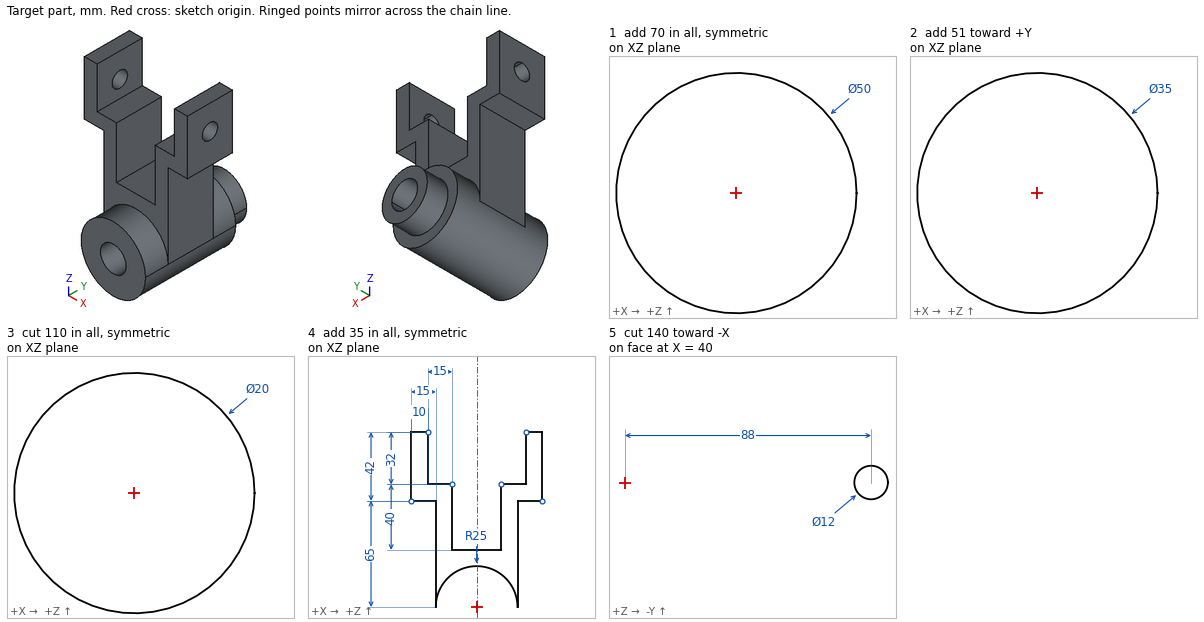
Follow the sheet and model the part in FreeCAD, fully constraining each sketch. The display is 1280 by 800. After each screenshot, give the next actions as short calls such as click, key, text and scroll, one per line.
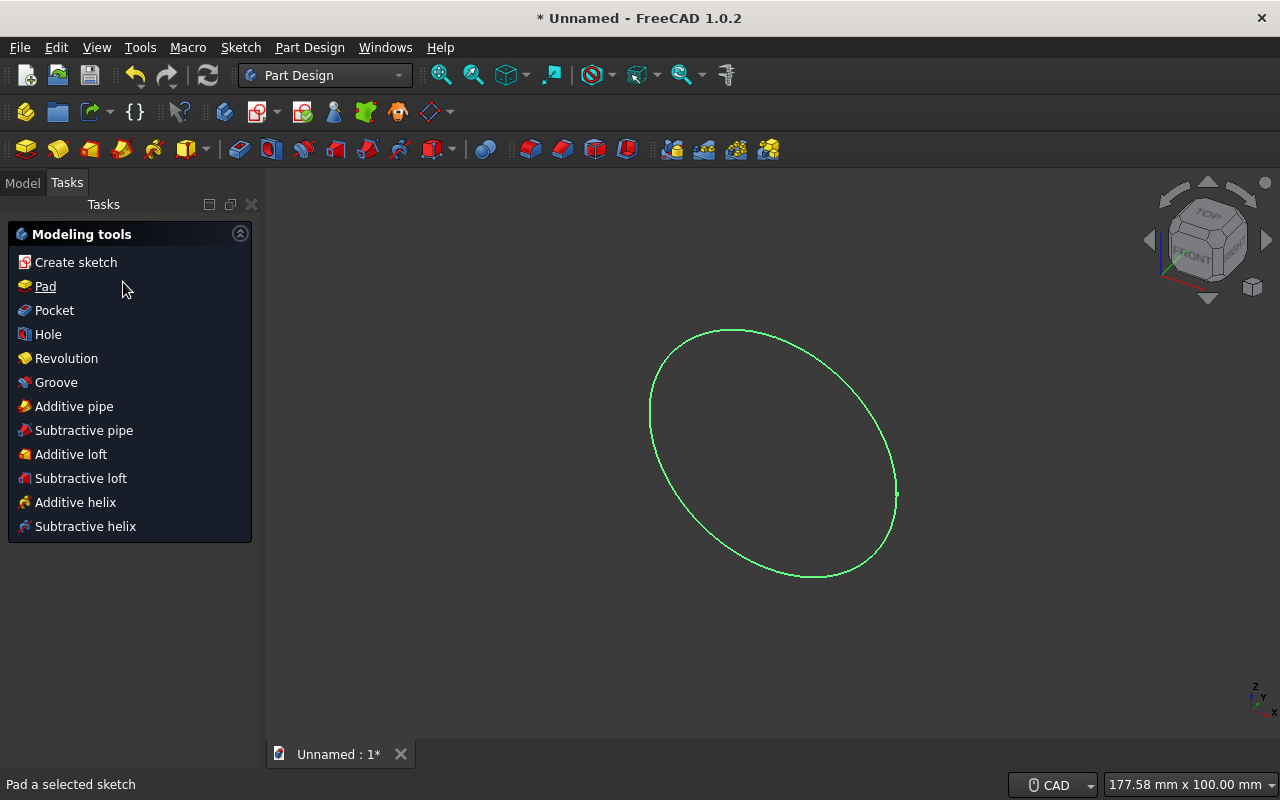
click(26, 150)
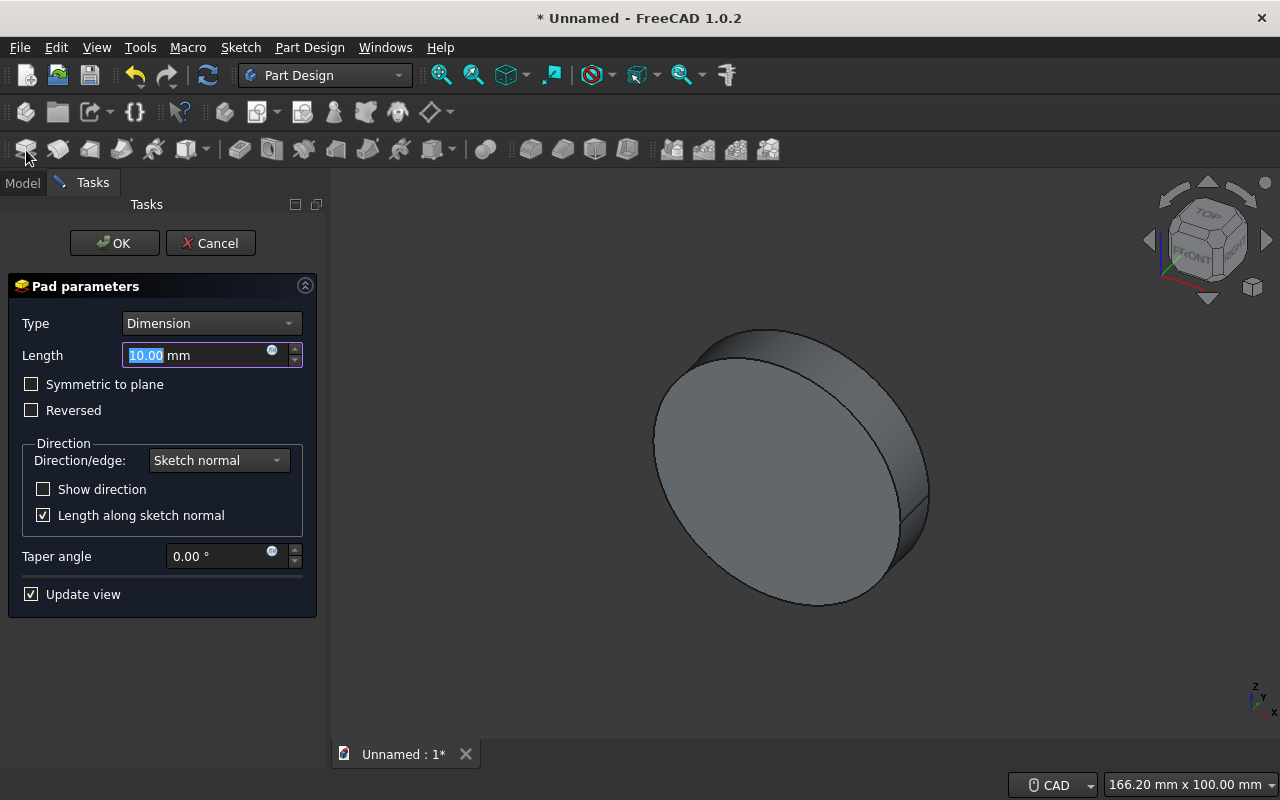
text(70)
key(Tab)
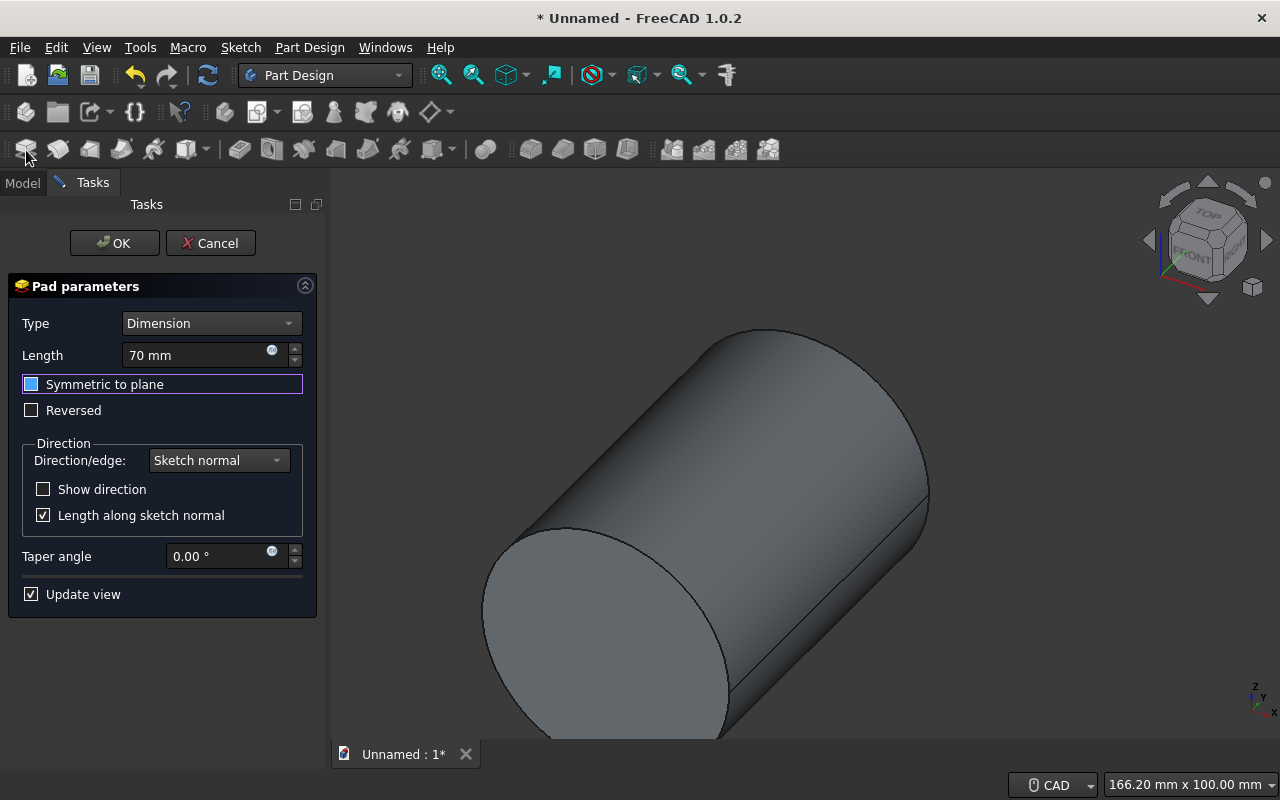
click(30, 384)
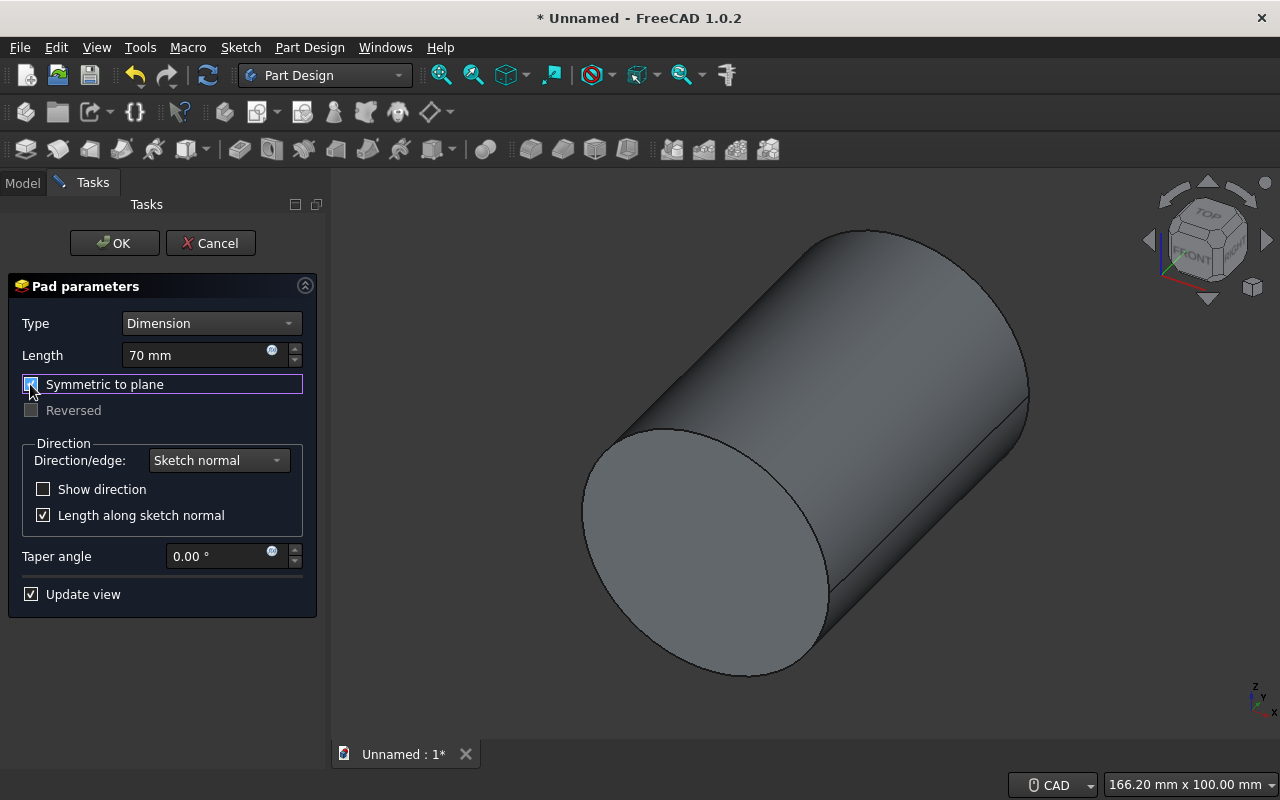
click(115, 243)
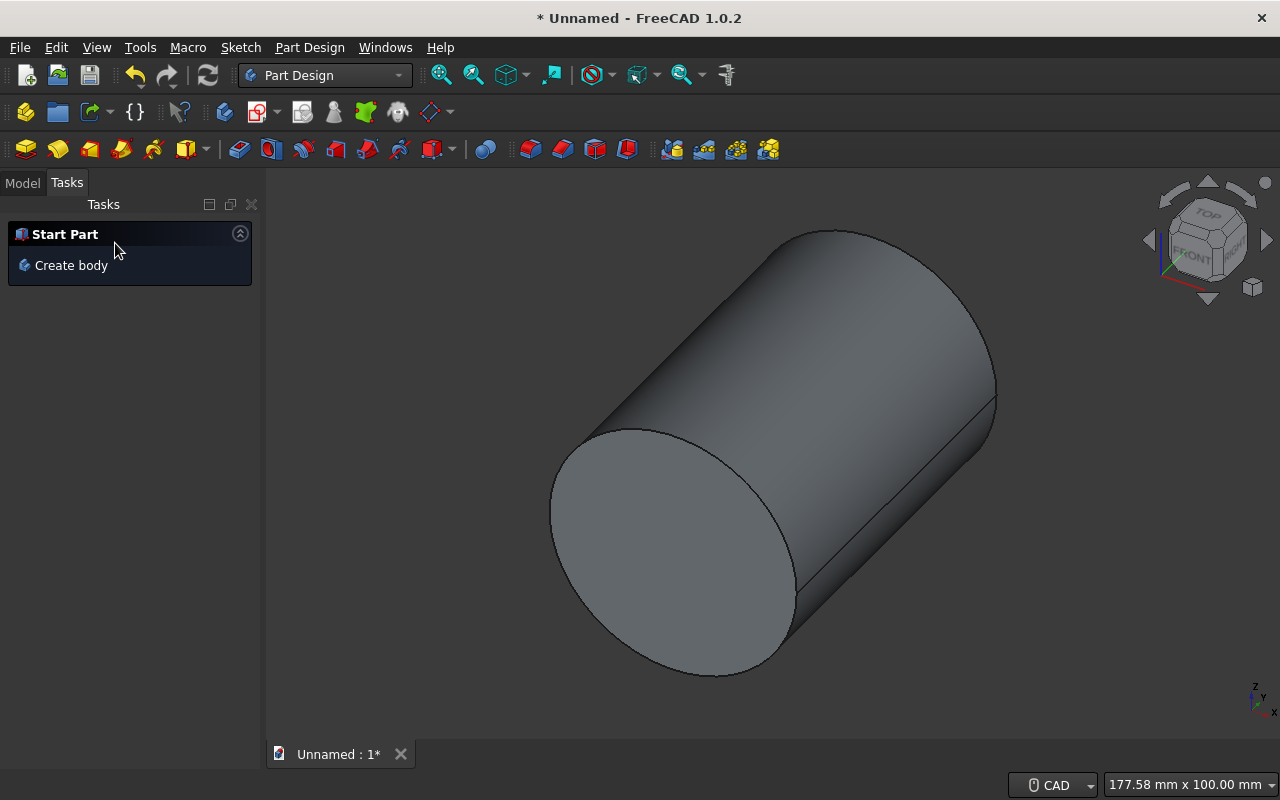
click(258, 112)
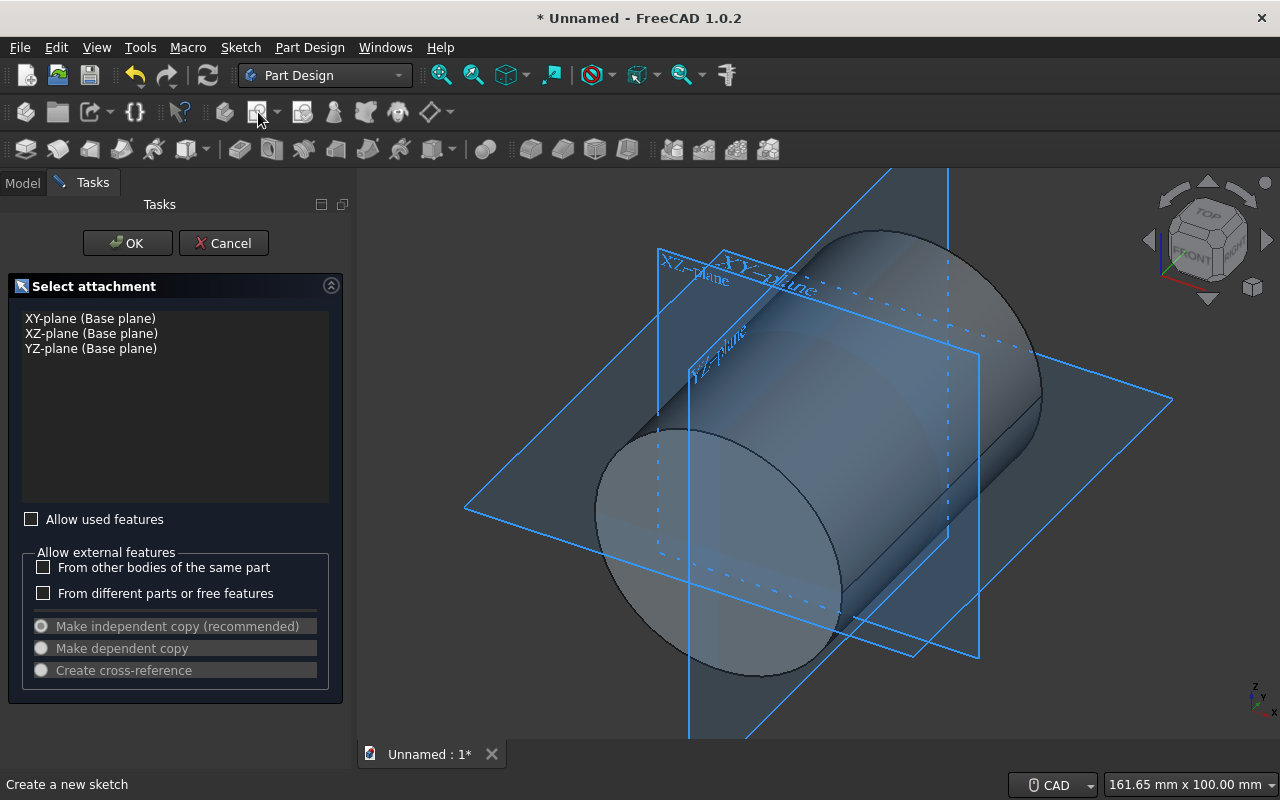
click(82, 334)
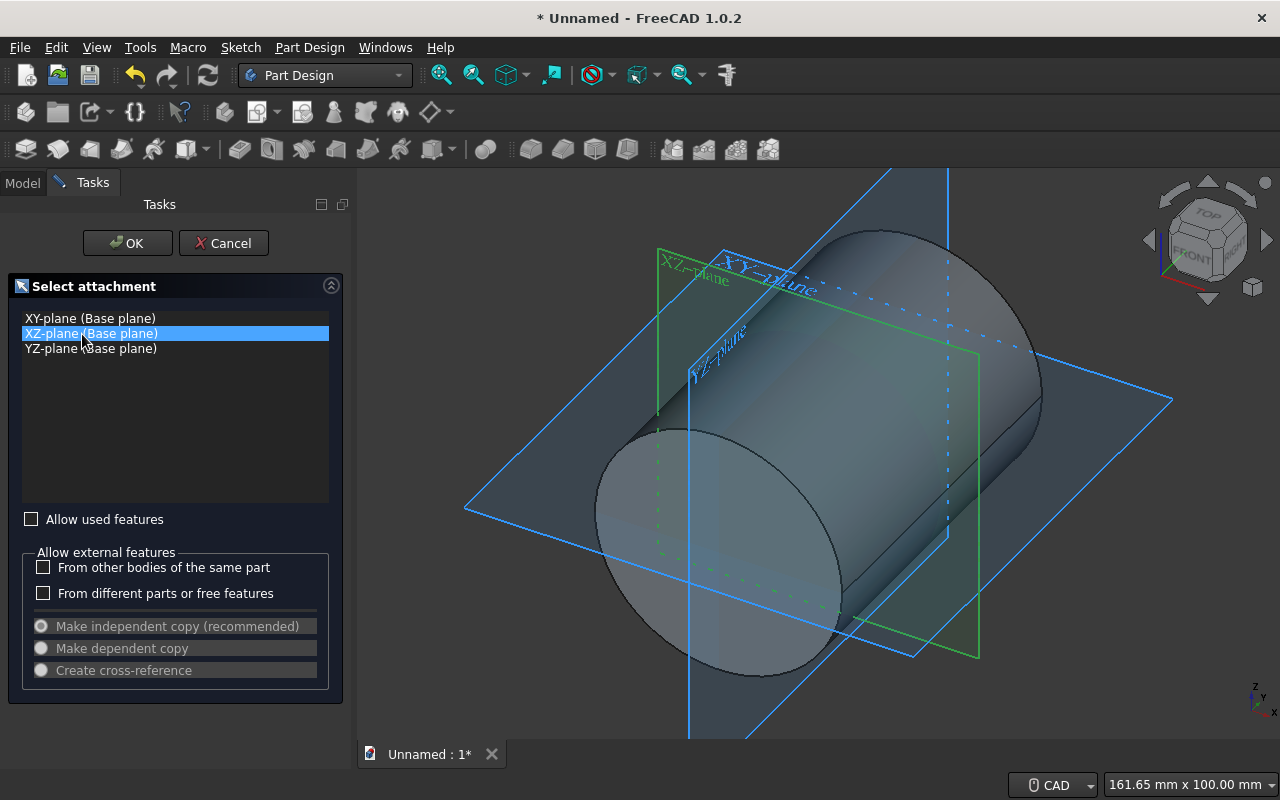
click(128, 243)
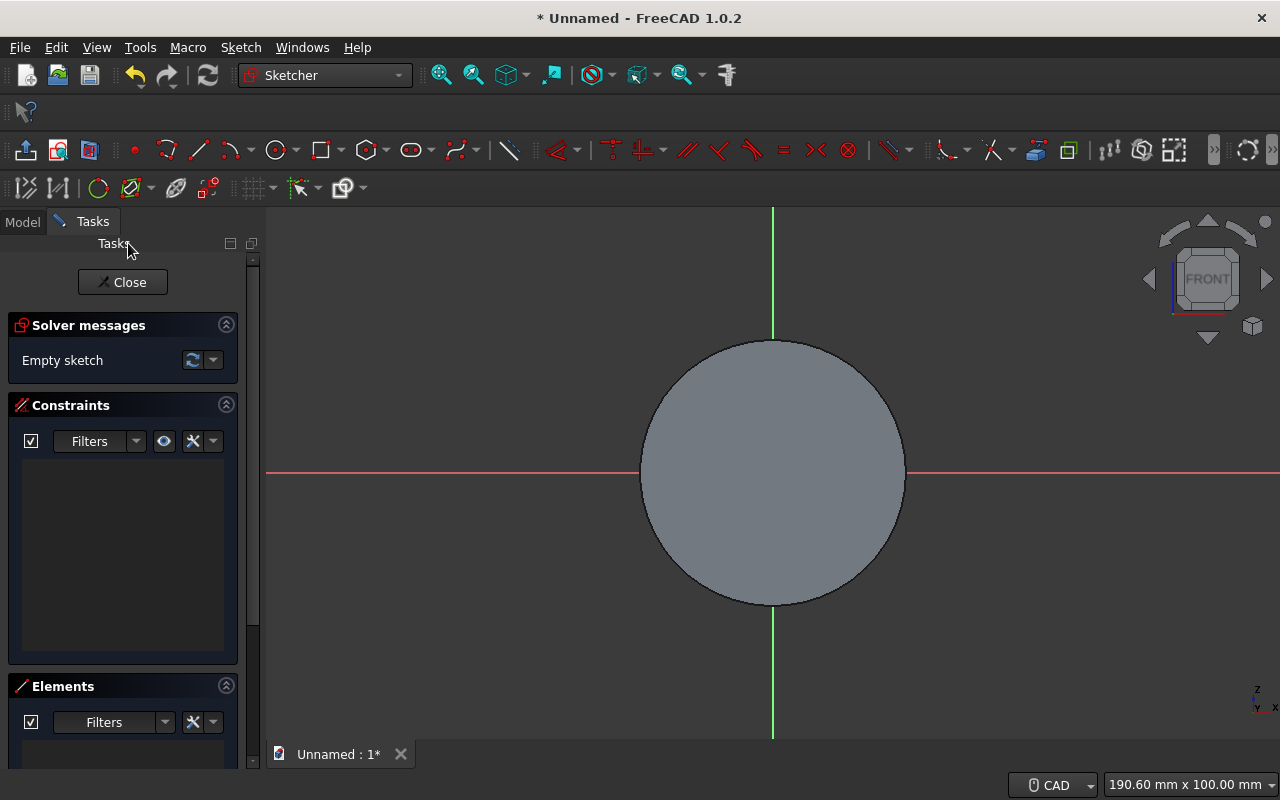
key(q)
key(s)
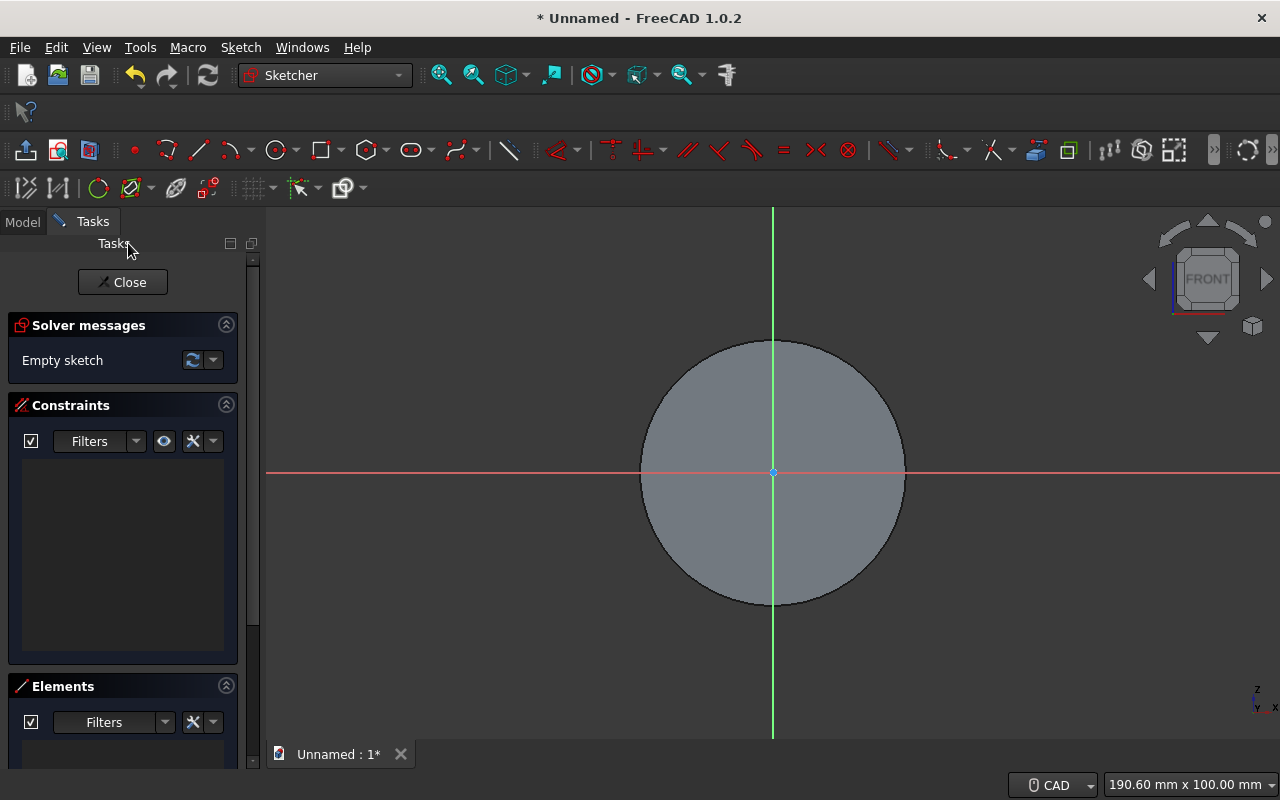
scroll(856, 473, up, 3)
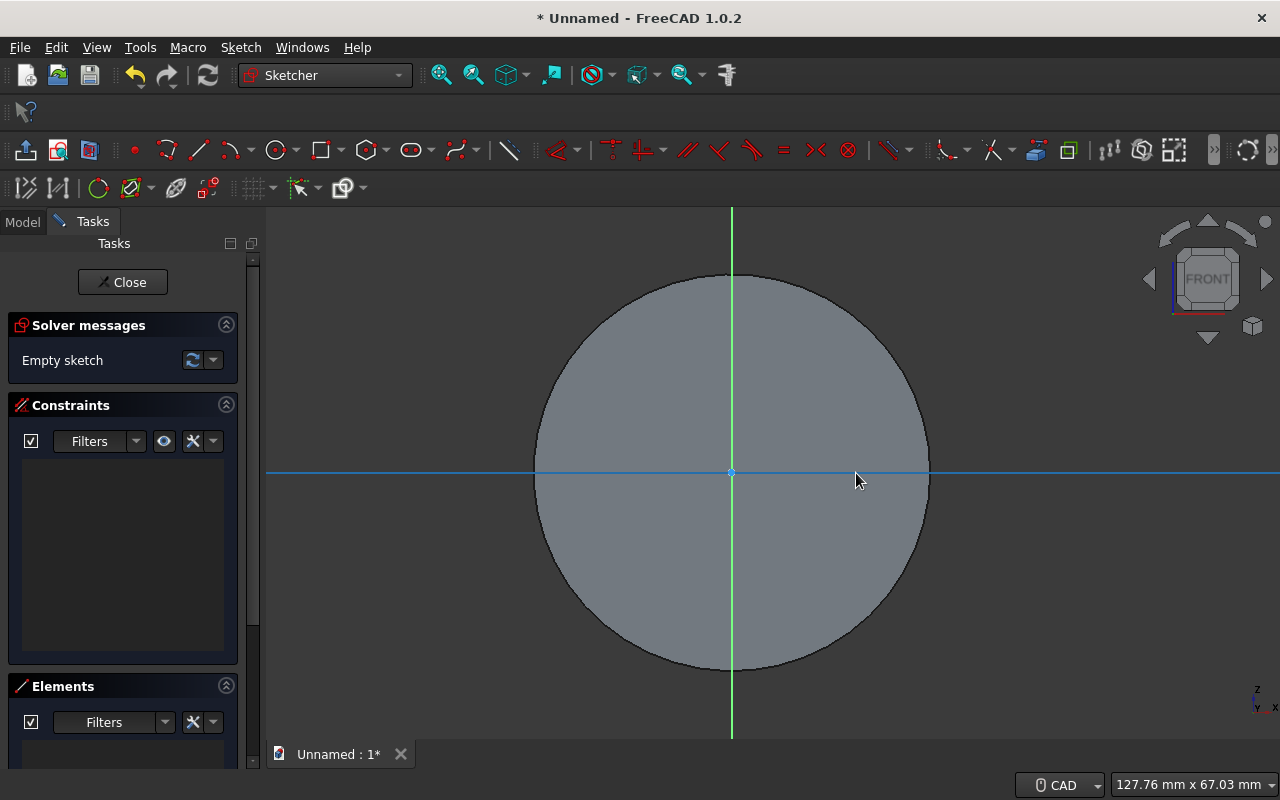
key(g)
key(c)